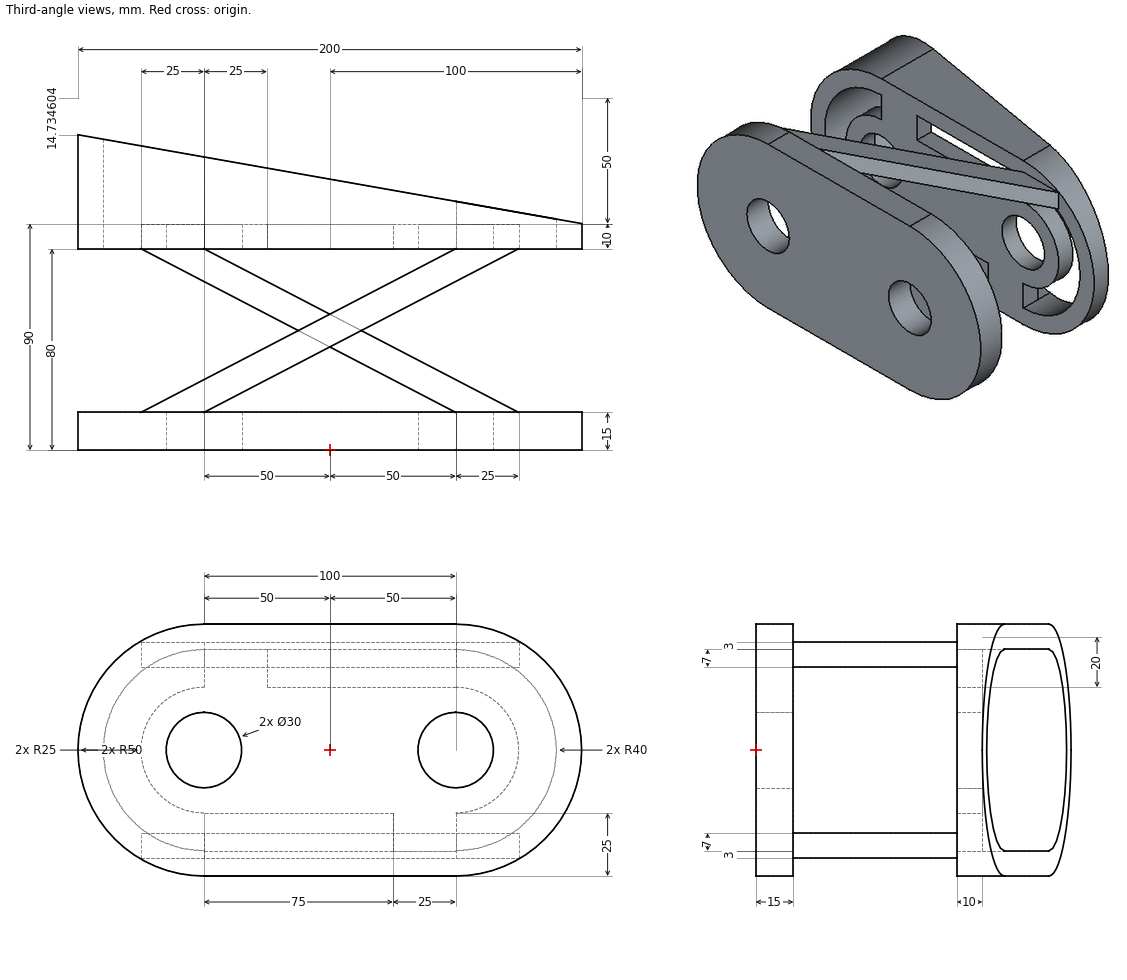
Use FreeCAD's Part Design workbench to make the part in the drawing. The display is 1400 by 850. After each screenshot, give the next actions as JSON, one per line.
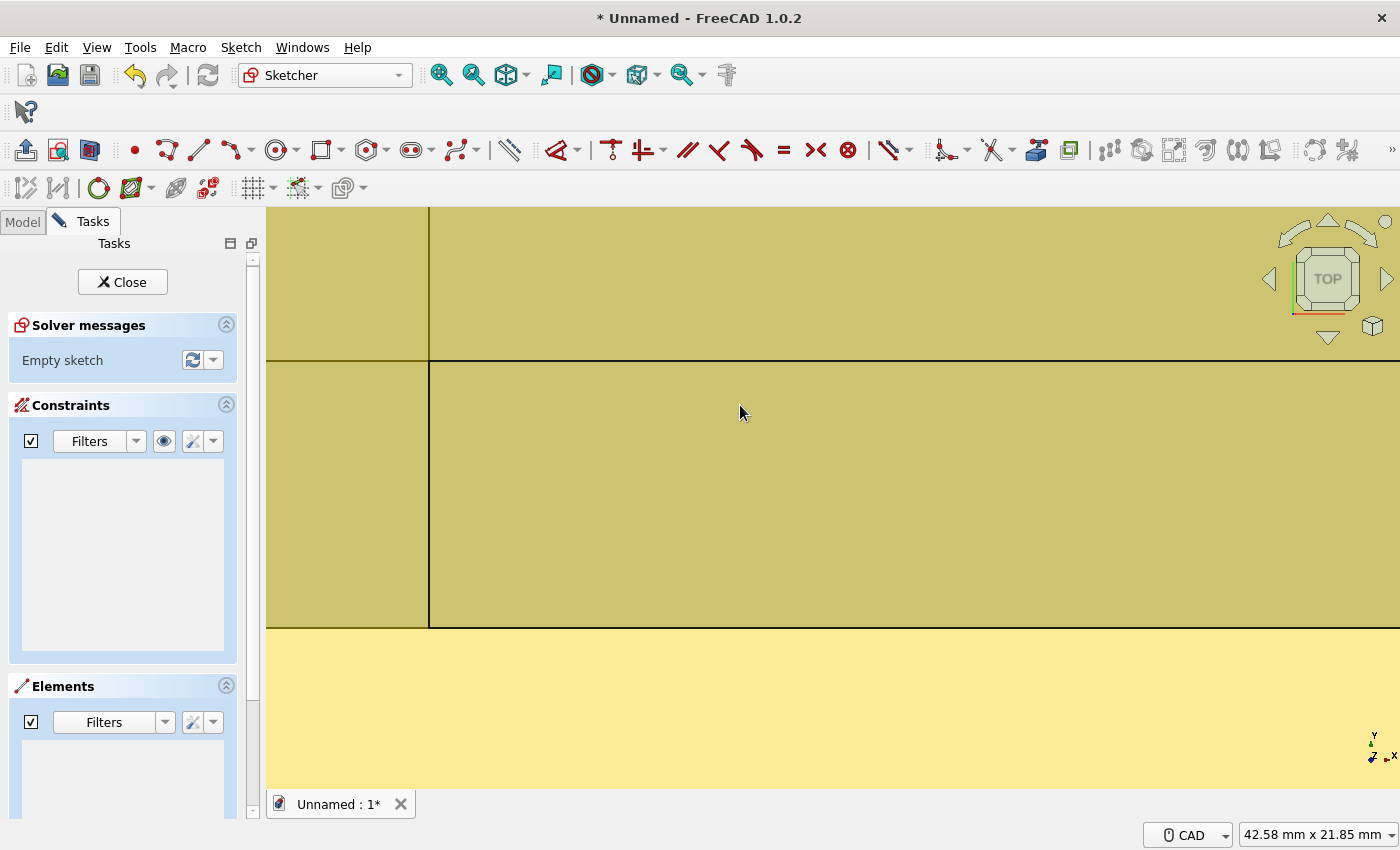
{"action": "left_click", "coordinate": [322, 150]}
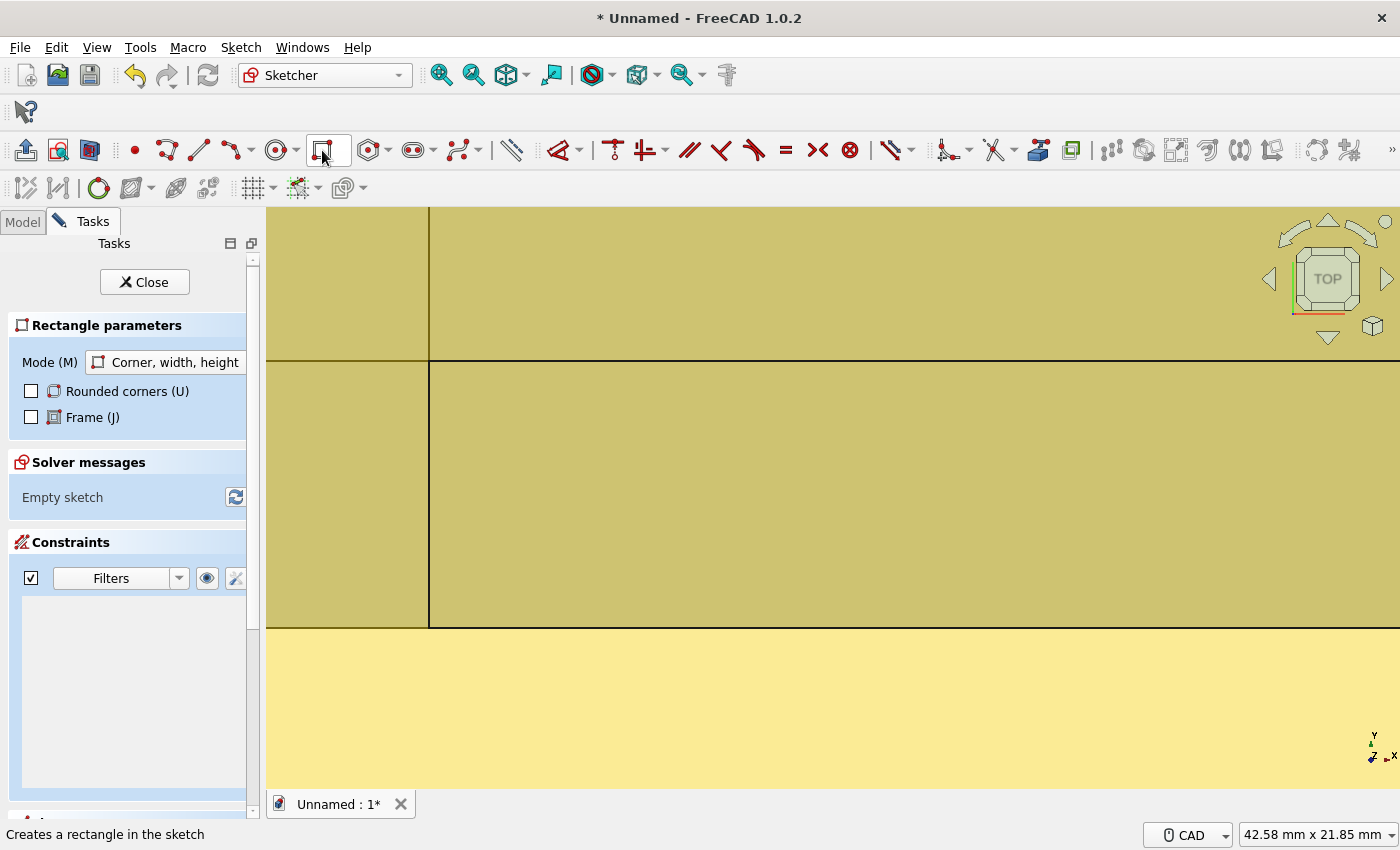
{"action": "left_click", "coordinate": [429, 361]}
{"action": "left_click", "coordinate": [1095, 628]}
{"action": "key", "text": "Escape"}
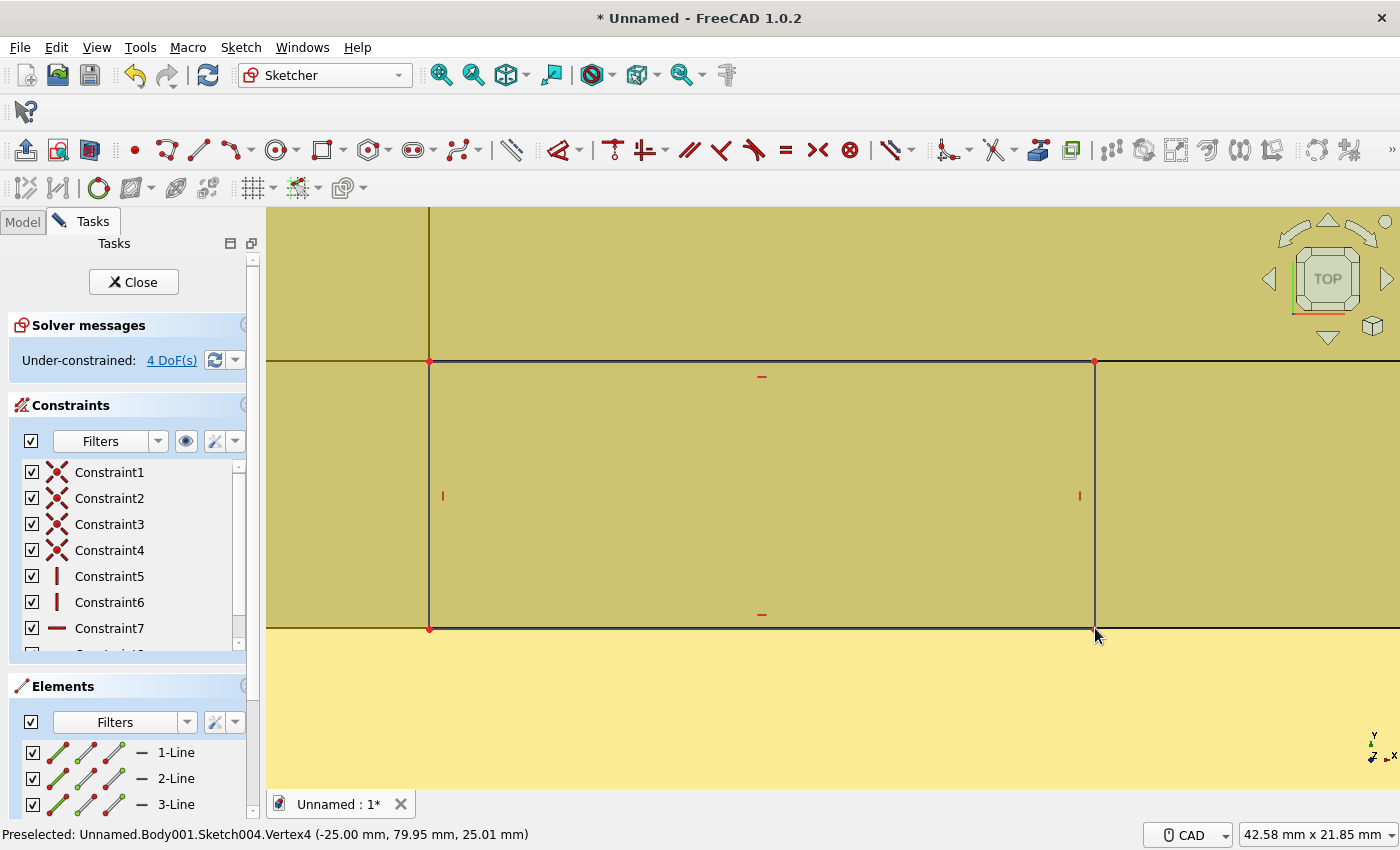
{"action": "left_click", "coordinate": [558, 150]}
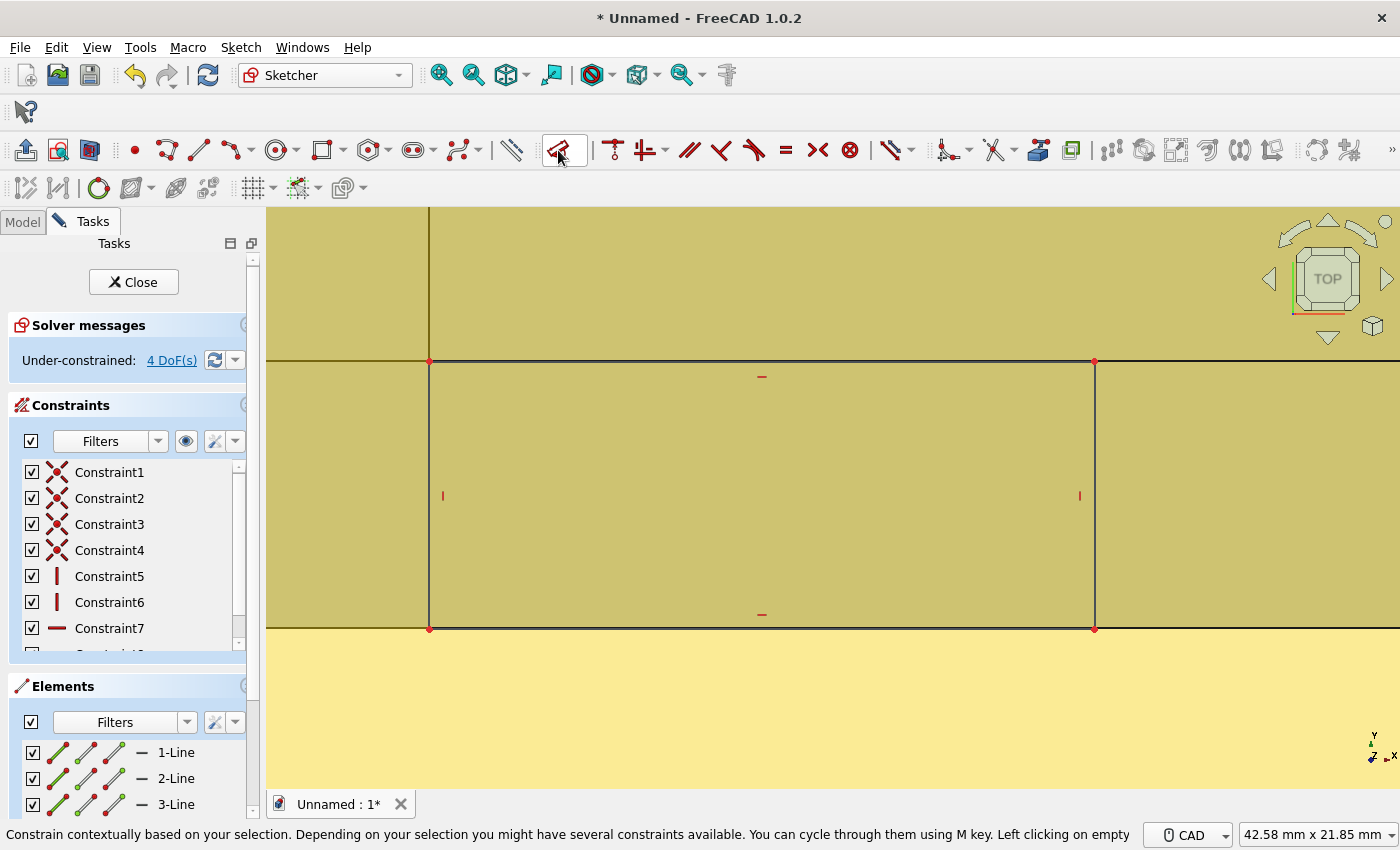
{"action": "left_click", "coordinate": [429, 442]}
{"action": "left_click", "coordinate": [395, 496]}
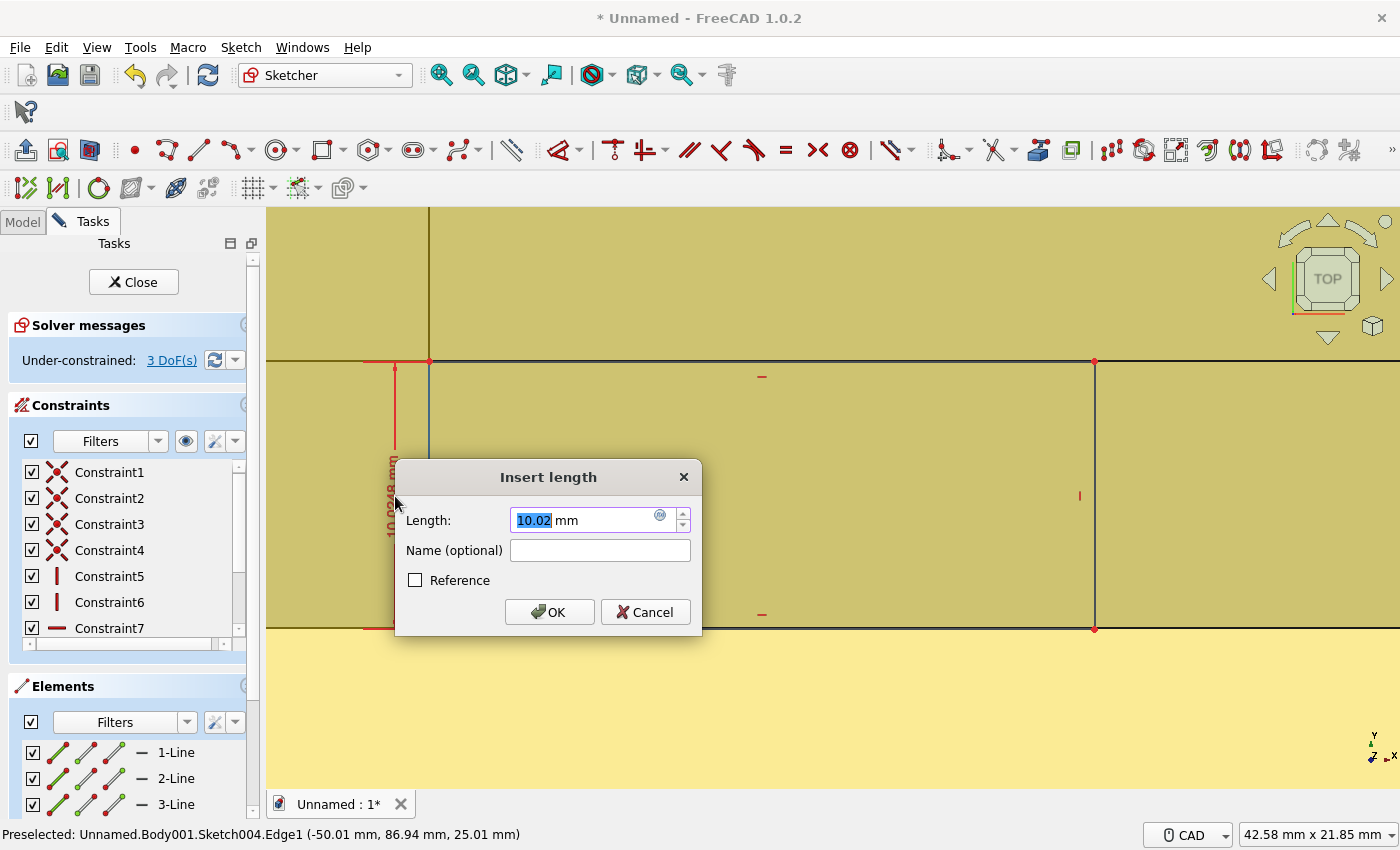
{"action": "type", "text": "10"}
{"action": "key", "text": "Return"}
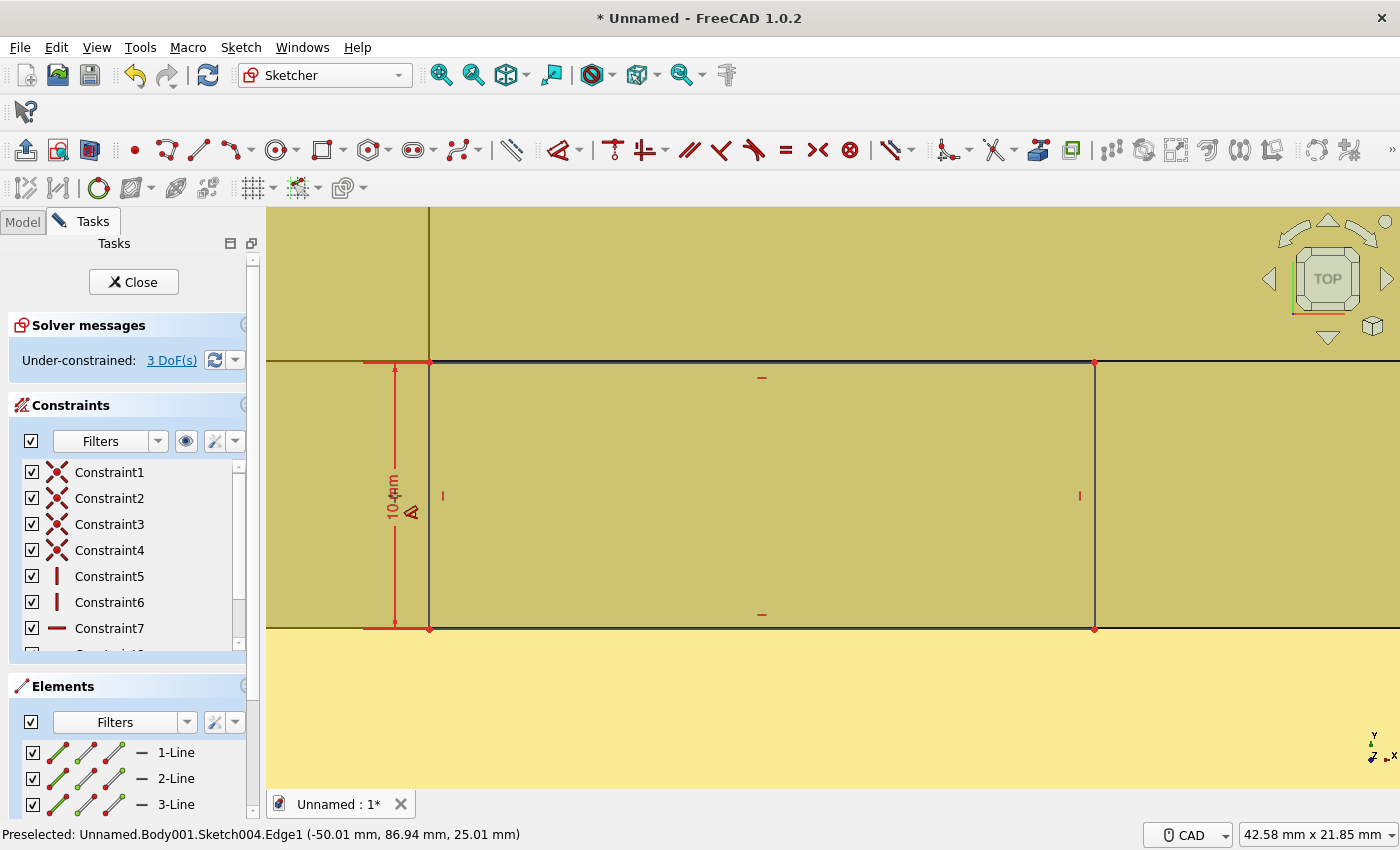
{"action": "left_click", "coordinate": [629, 629]}
{"action": "left_click", "coordinate": [762, 663]}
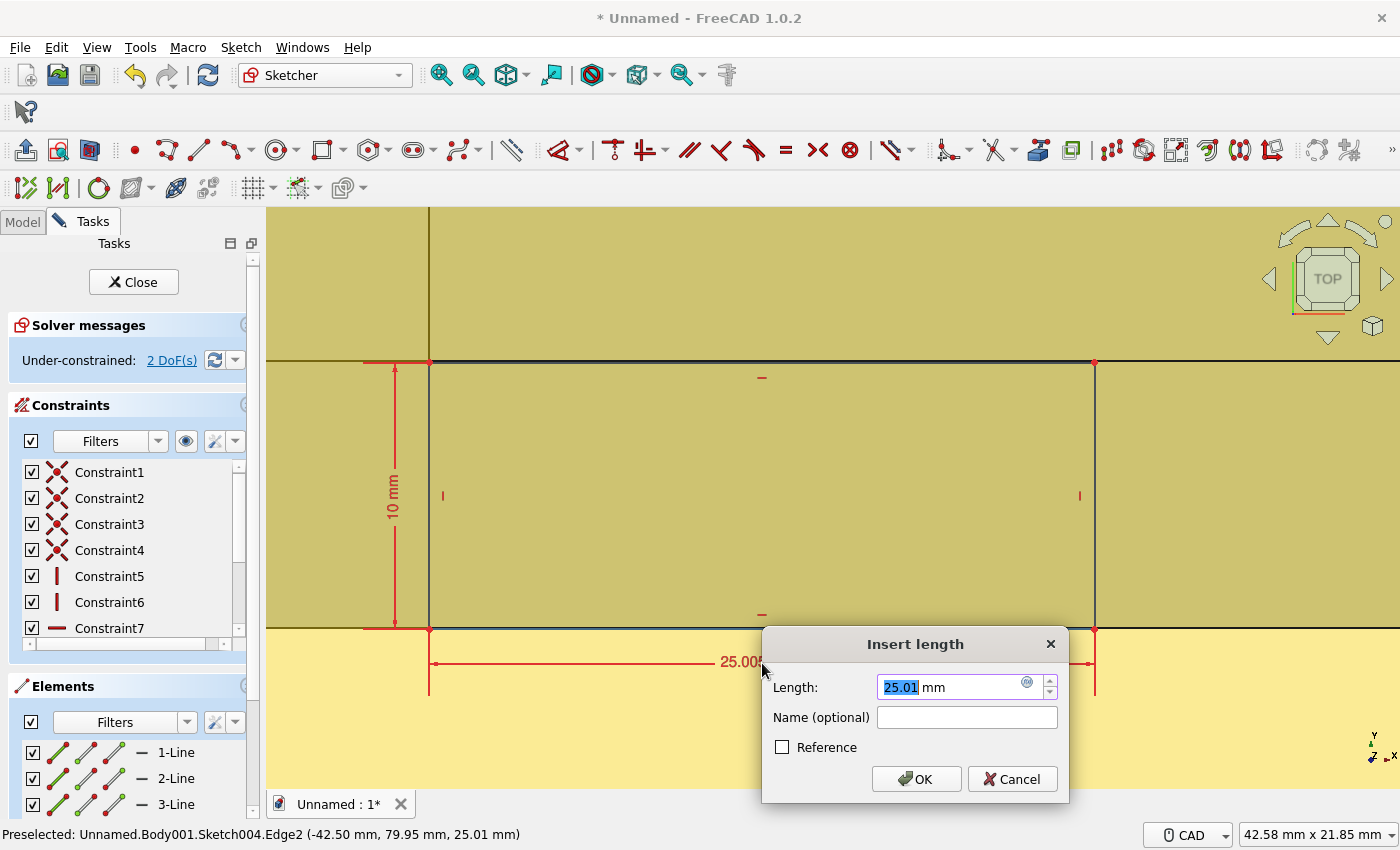
{"action": "type", "text": "25"}
{"action": "key", "text": "Return"}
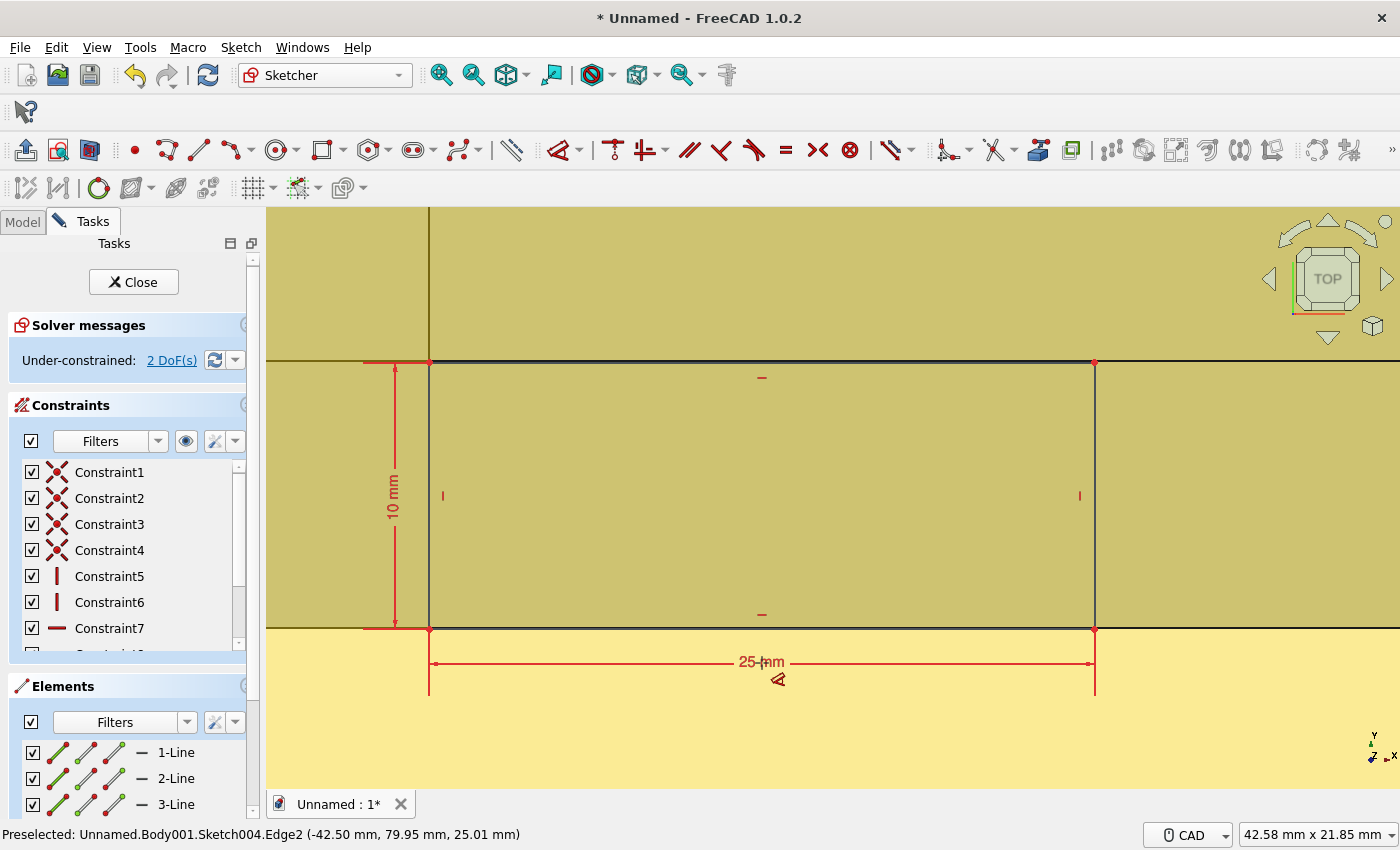
{"action": "left_click", "coordinate": [429, 363]}
{"action": "left_click", "coordinate": [832, 329]}